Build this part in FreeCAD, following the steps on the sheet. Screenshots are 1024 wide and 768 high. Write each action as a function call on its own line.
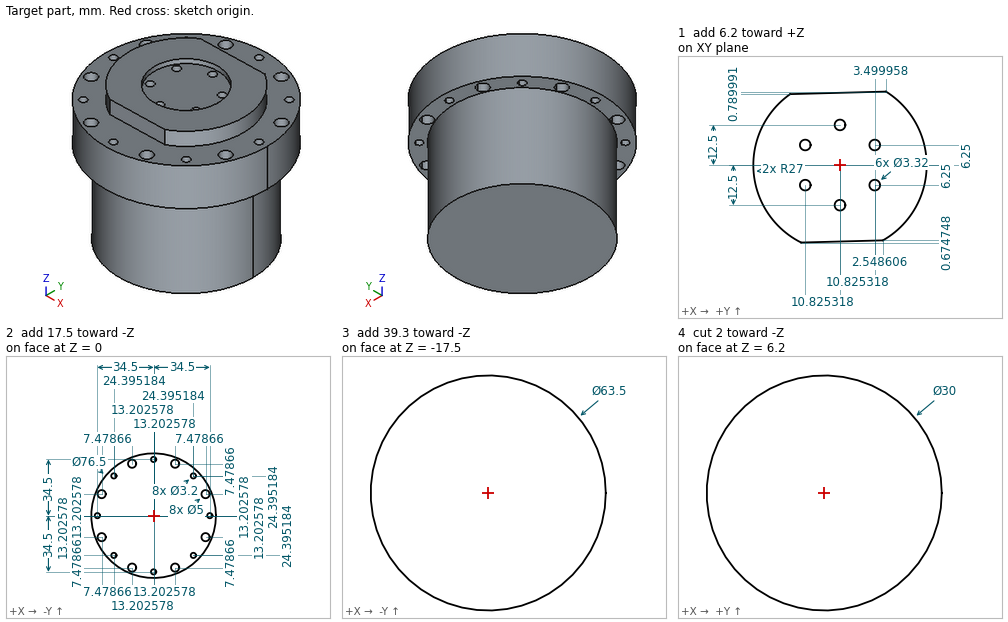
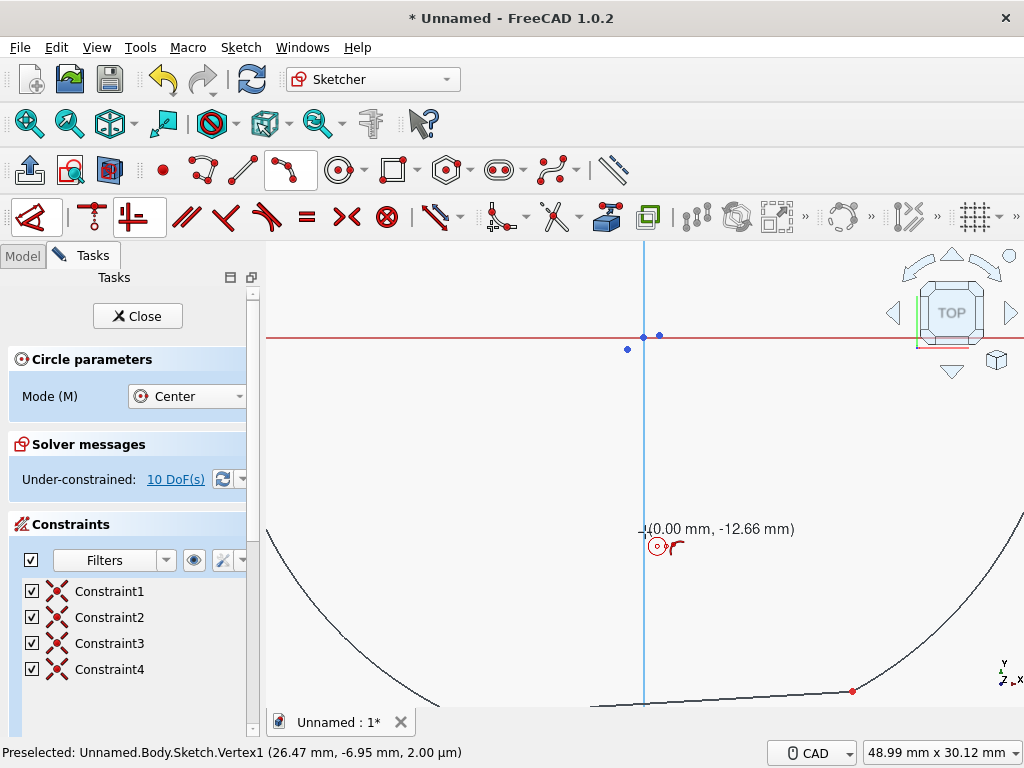
click(644, 531)
move(662, 513)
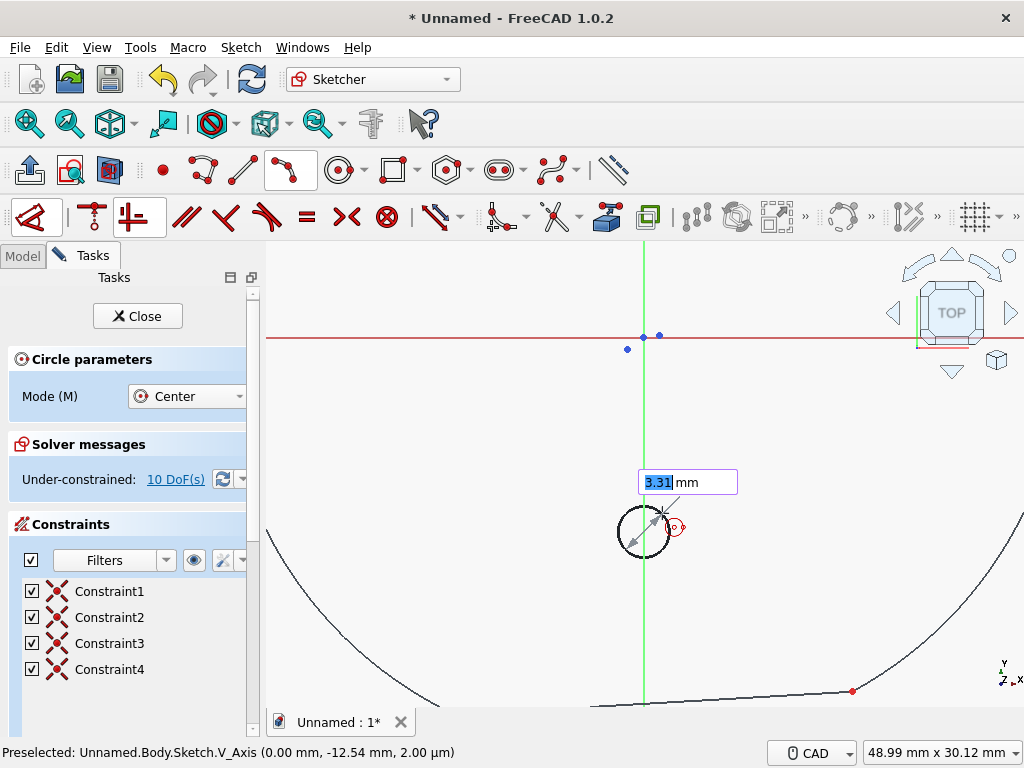
text(3.32)
key(Return)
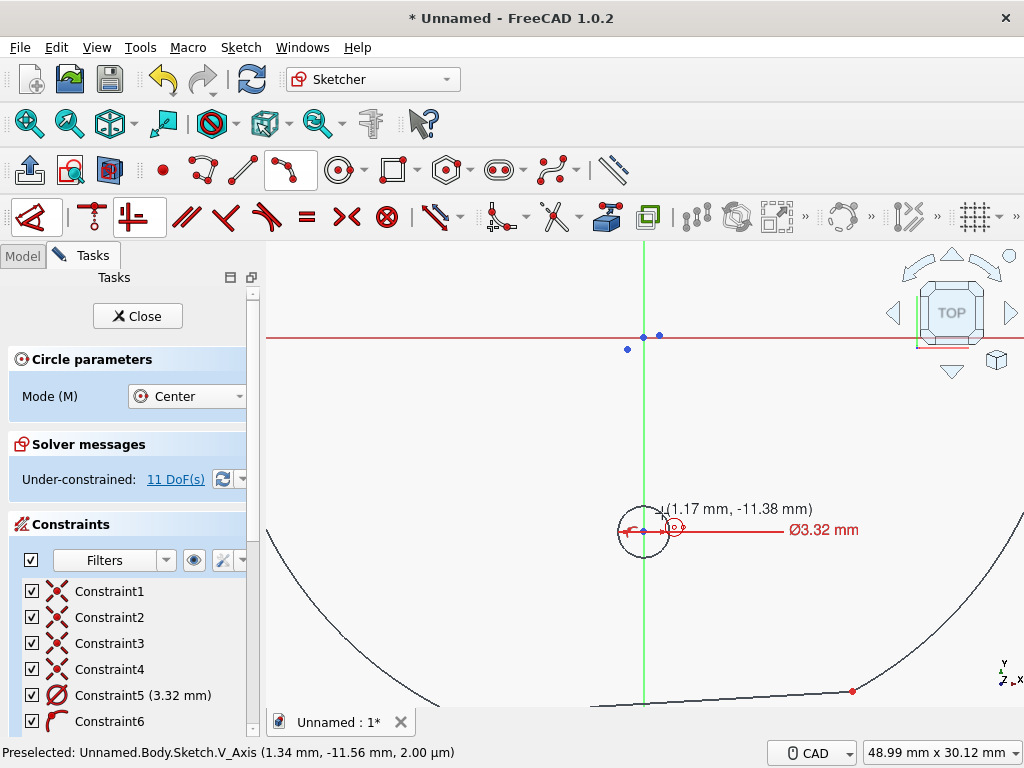
click(811, 435)
move(829, 417)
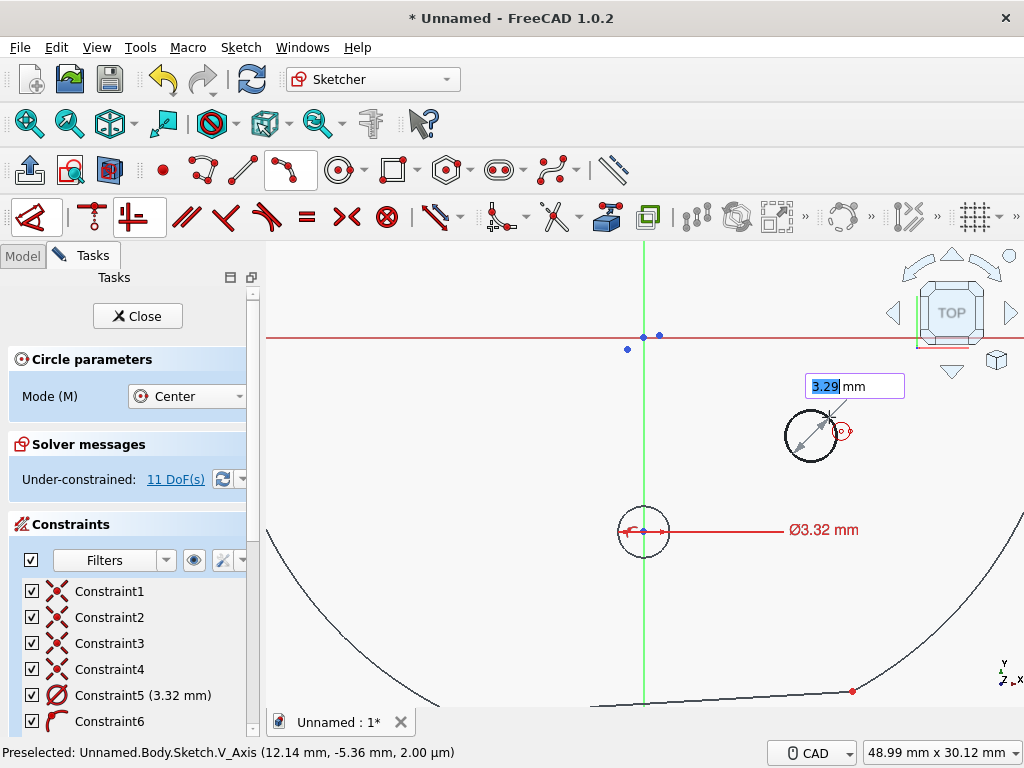
text(3.32)
key(Return)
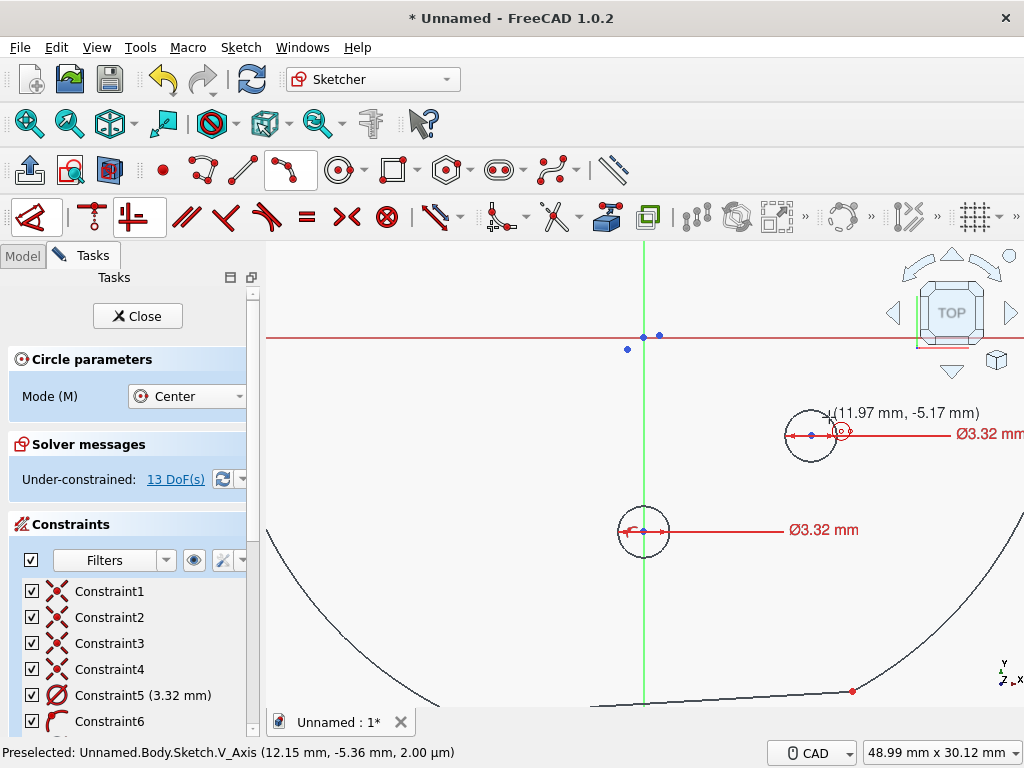
click(476, 435)
move(495, 417)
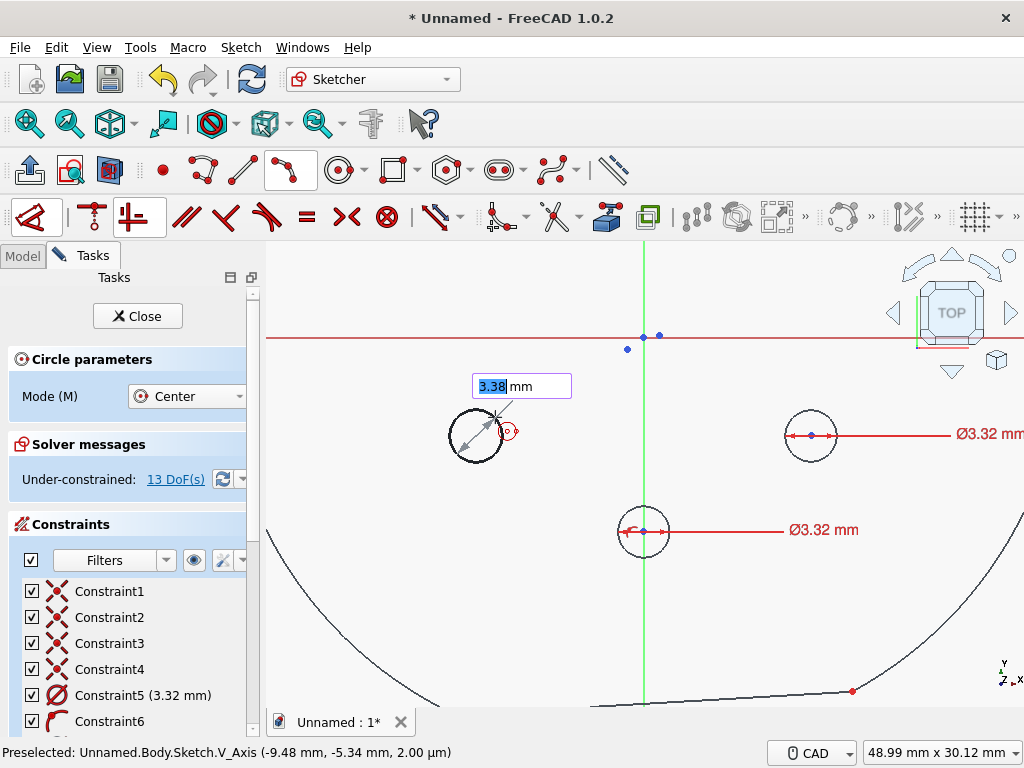
text(3.32)
key(Return)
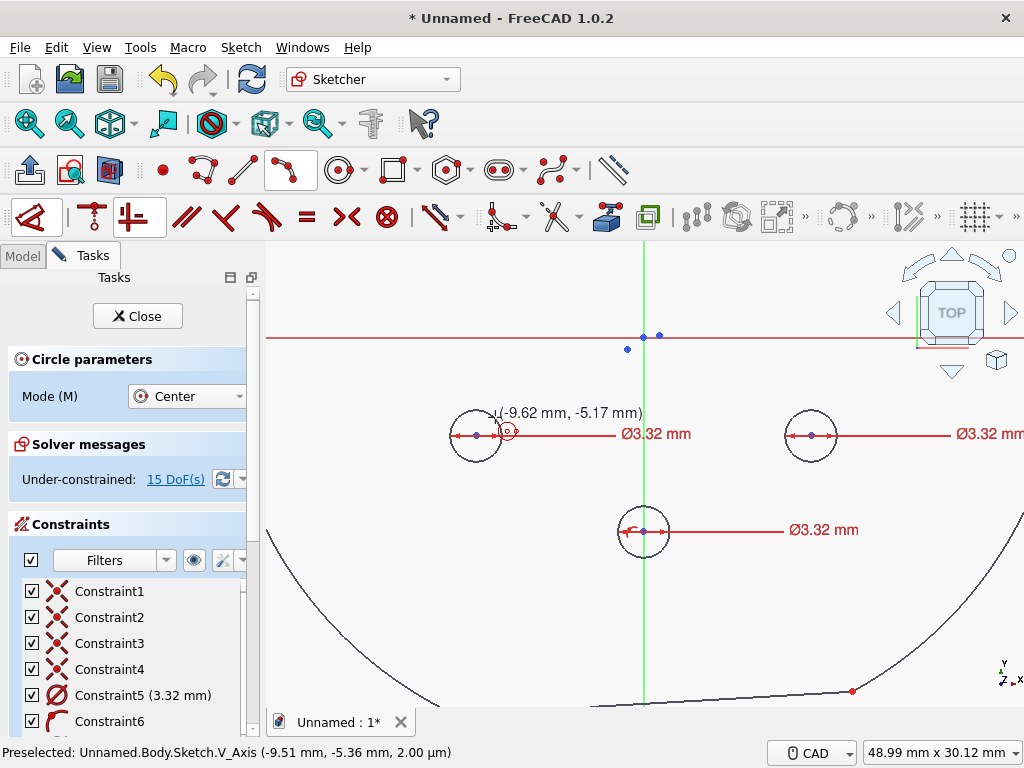
scroll(537, 548, down, 5)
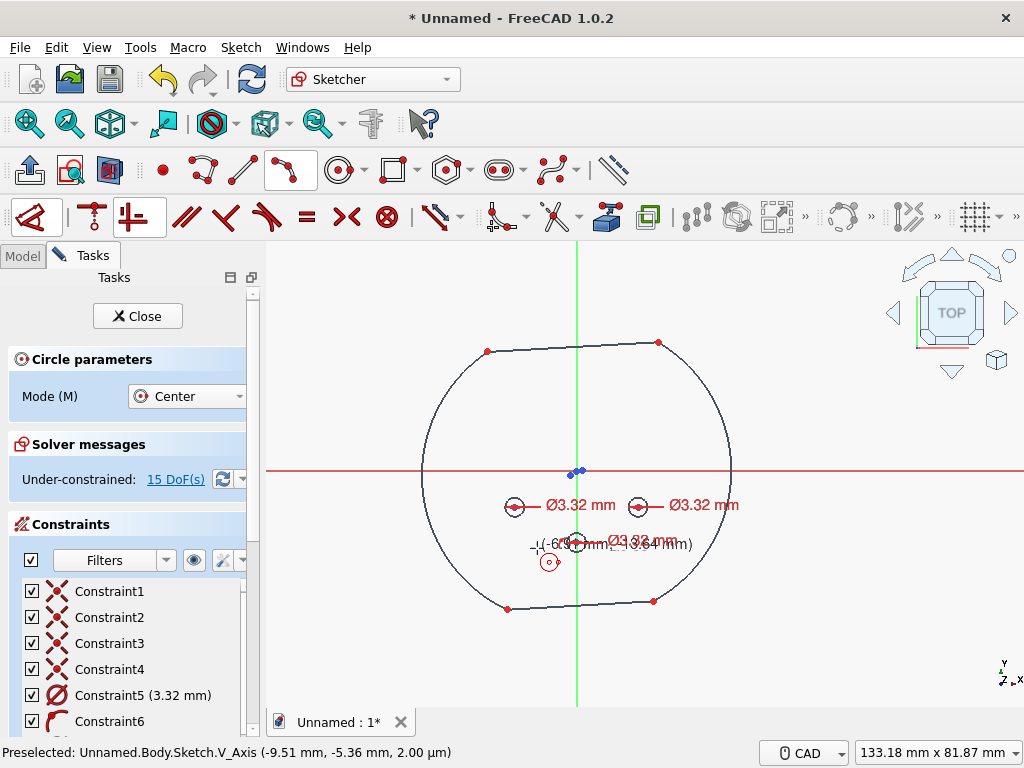
scroll(638, 436, up, 5)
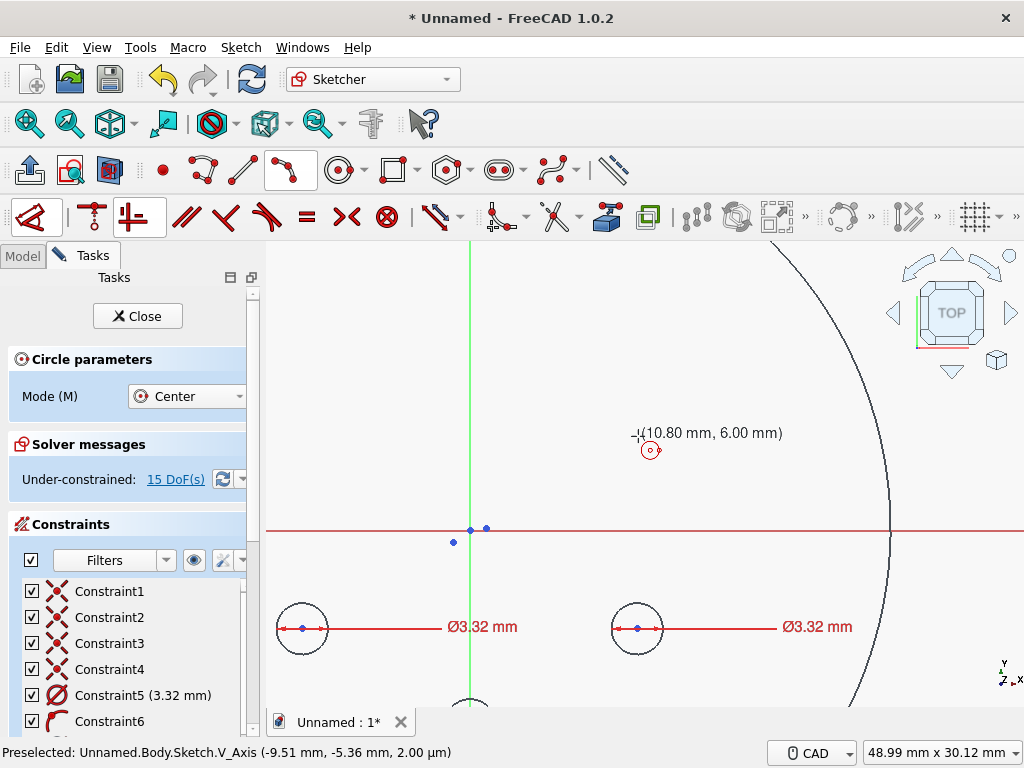
click(638, 434)
move(656, 416)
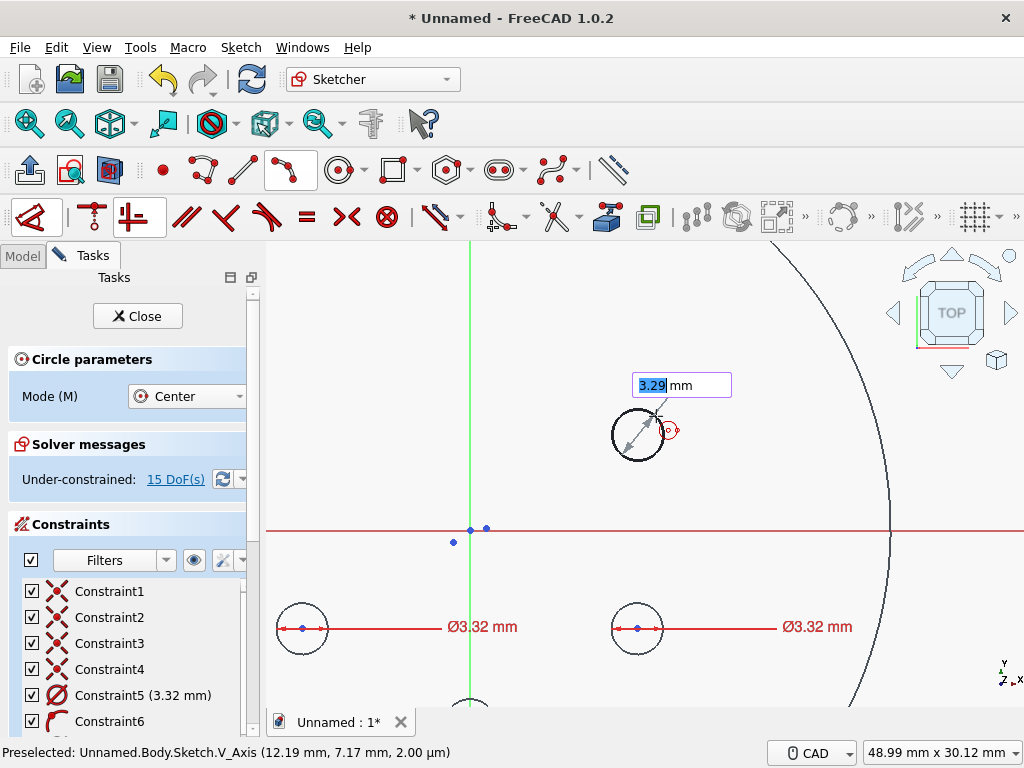
text(3.32)
key(Return)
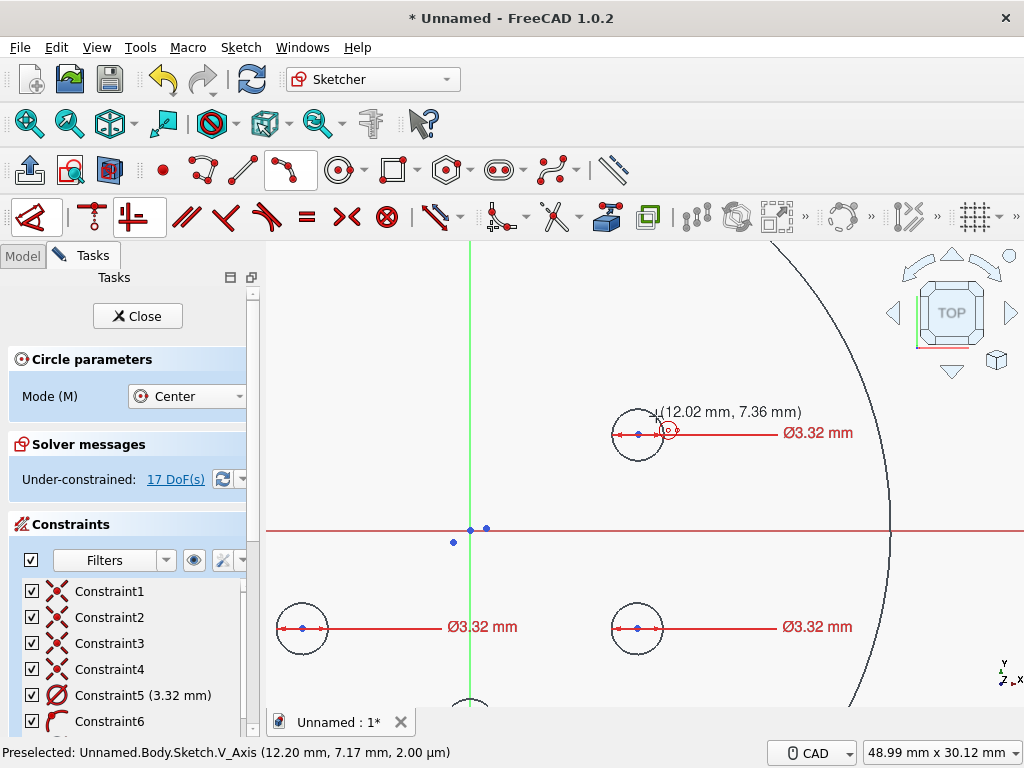
click(470, 337)
move(488, 319)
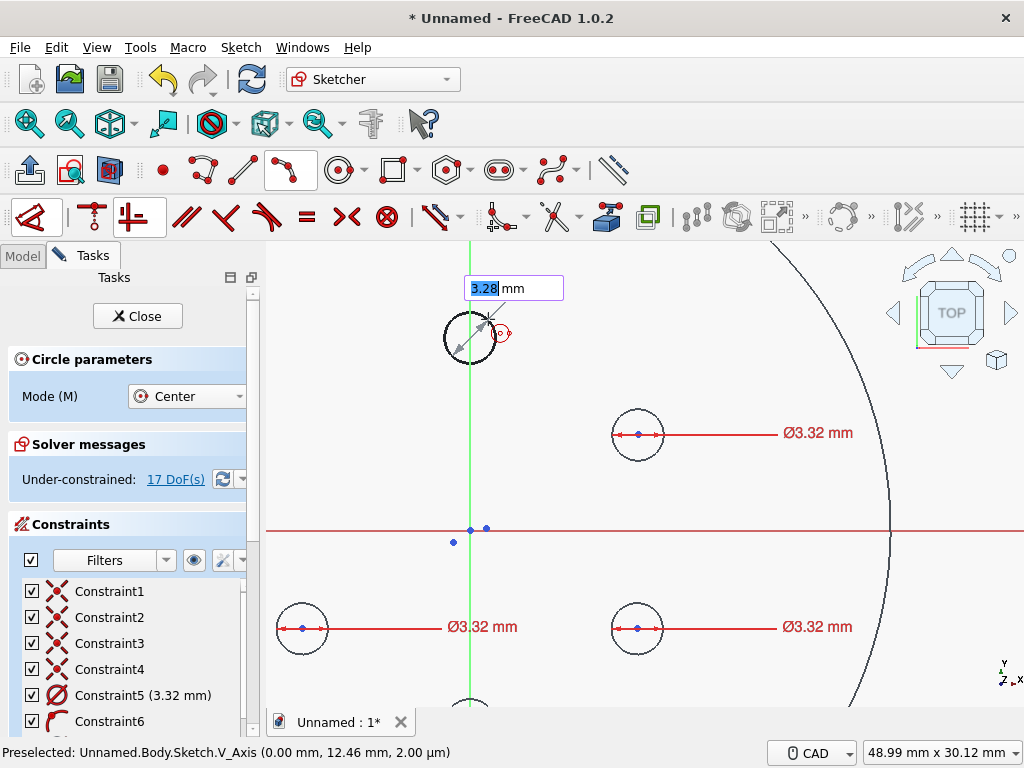
text(3.32)
key(Return)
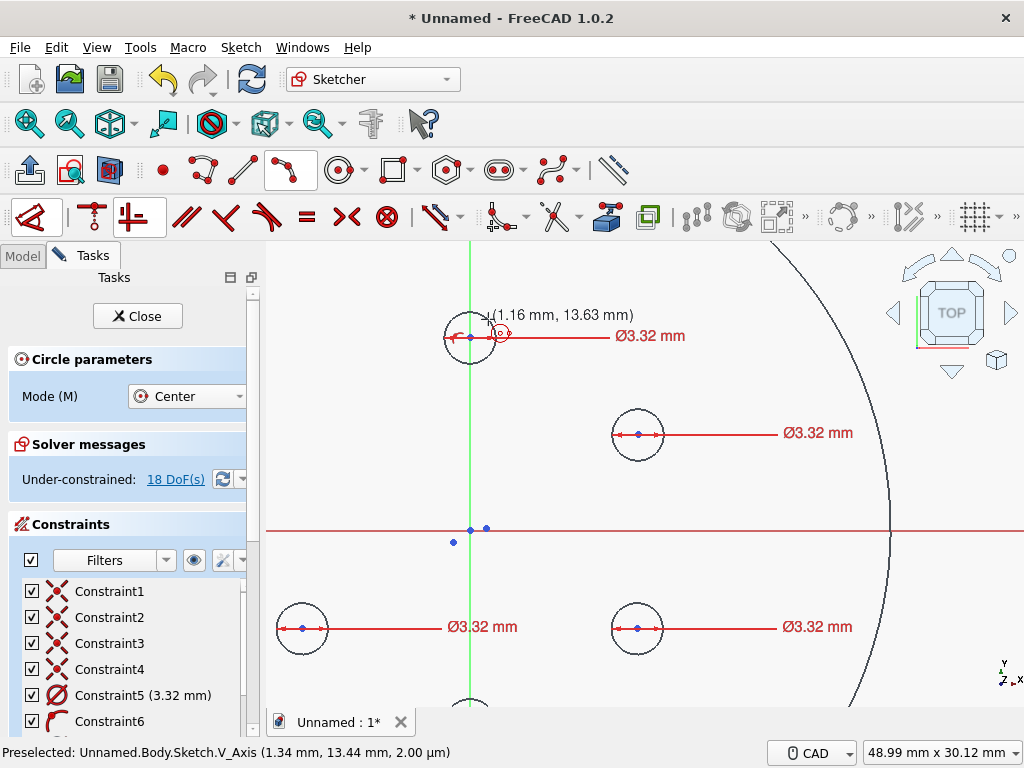
click(303, 434)
move(321, 416)